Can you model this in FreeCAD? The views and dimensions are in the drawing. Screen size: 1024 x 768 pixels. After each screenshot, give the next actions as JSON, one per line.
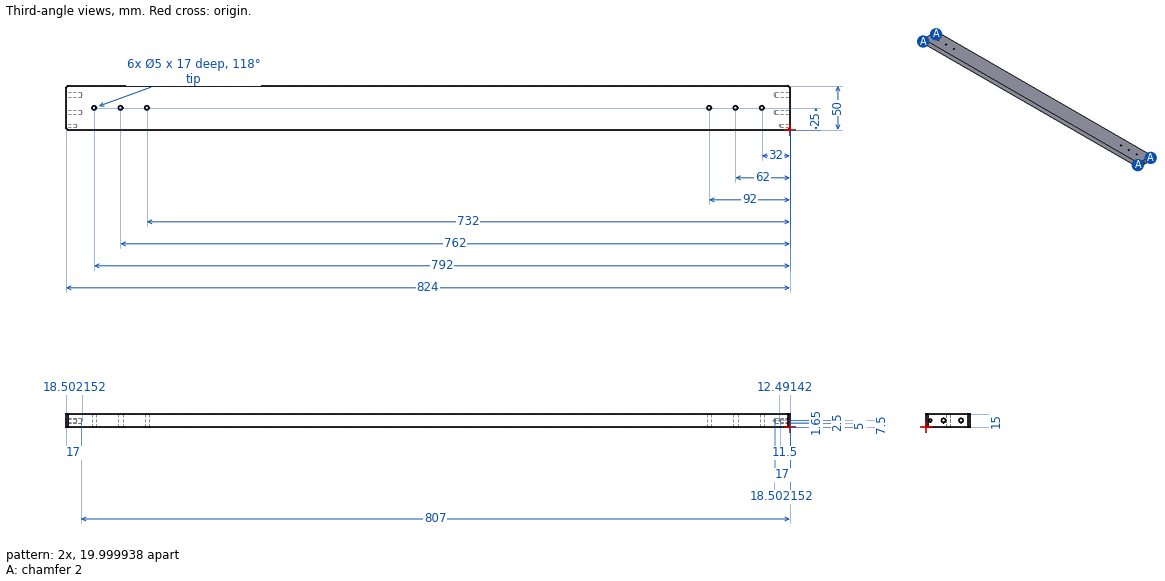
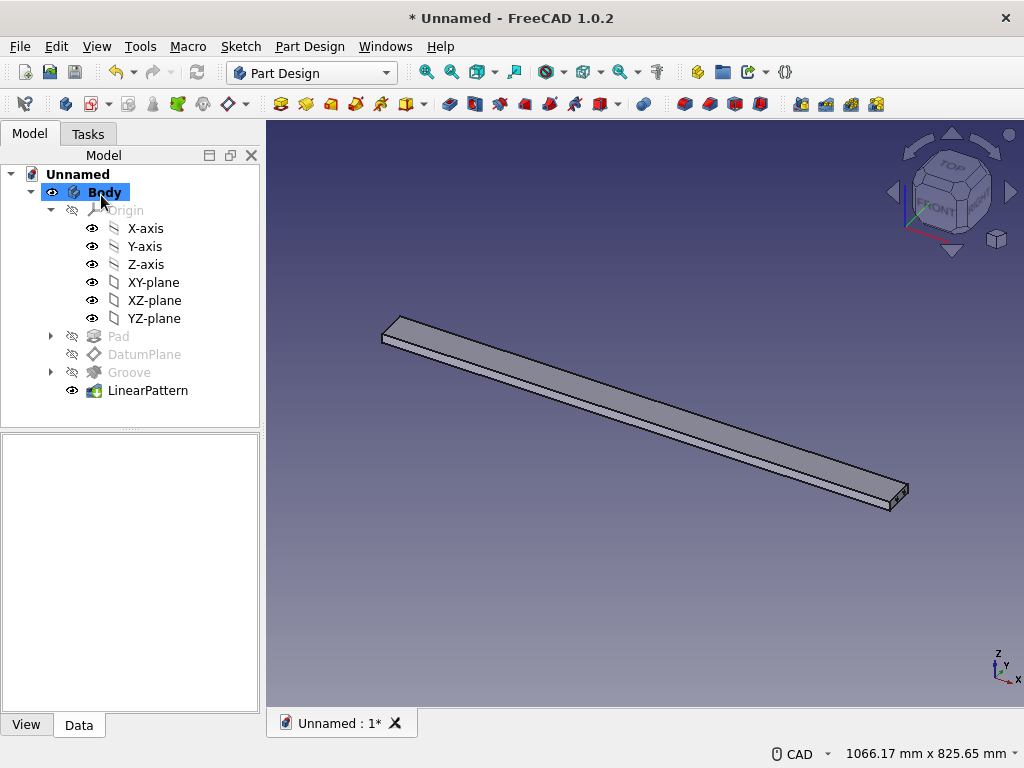
{"action": "left_click", "coordinate": [137, 300]}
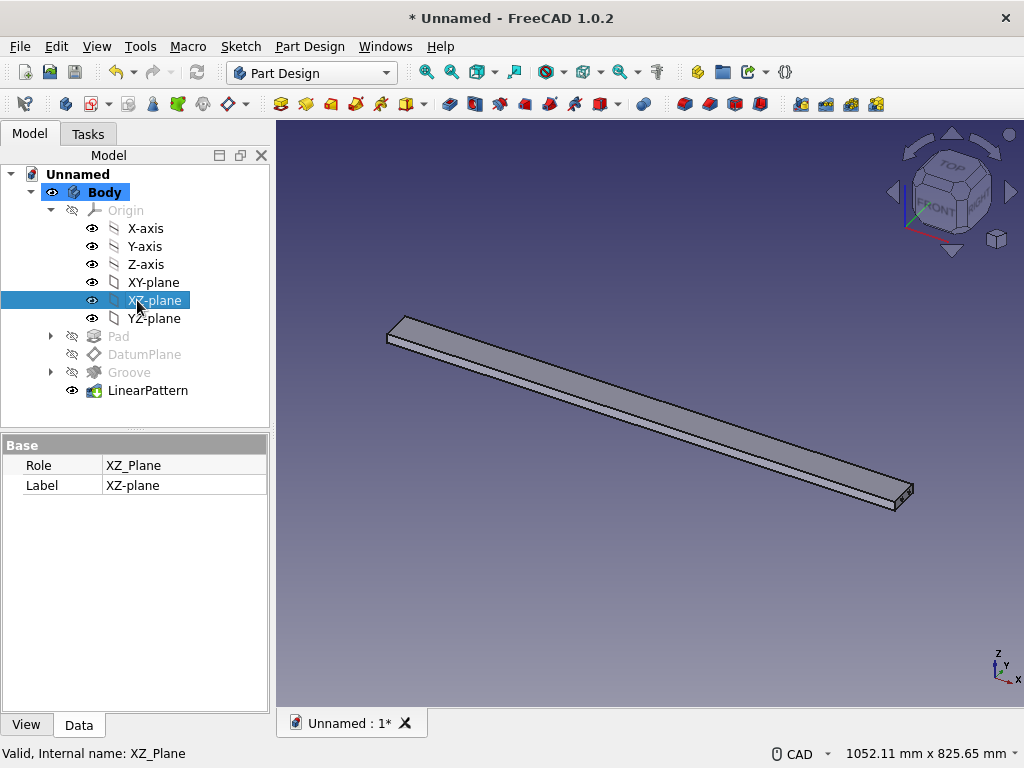
{"action": "left_click", "coordinate": [228, 104]}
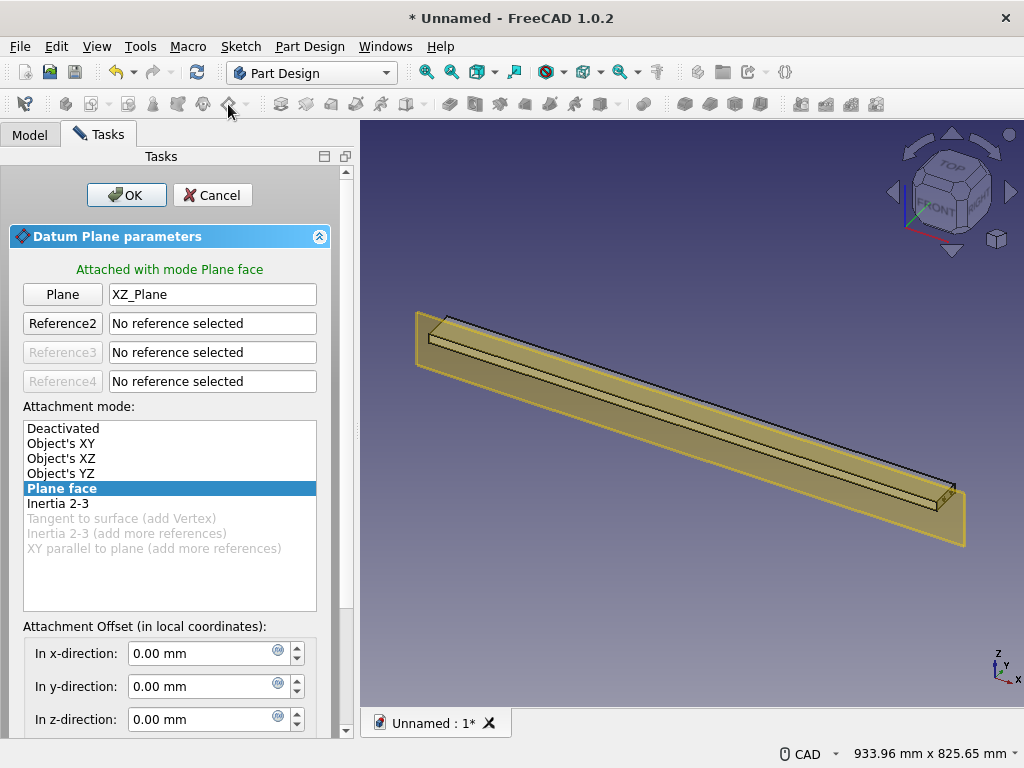
{"action": "triple_click", "coordinate": [210, 720]}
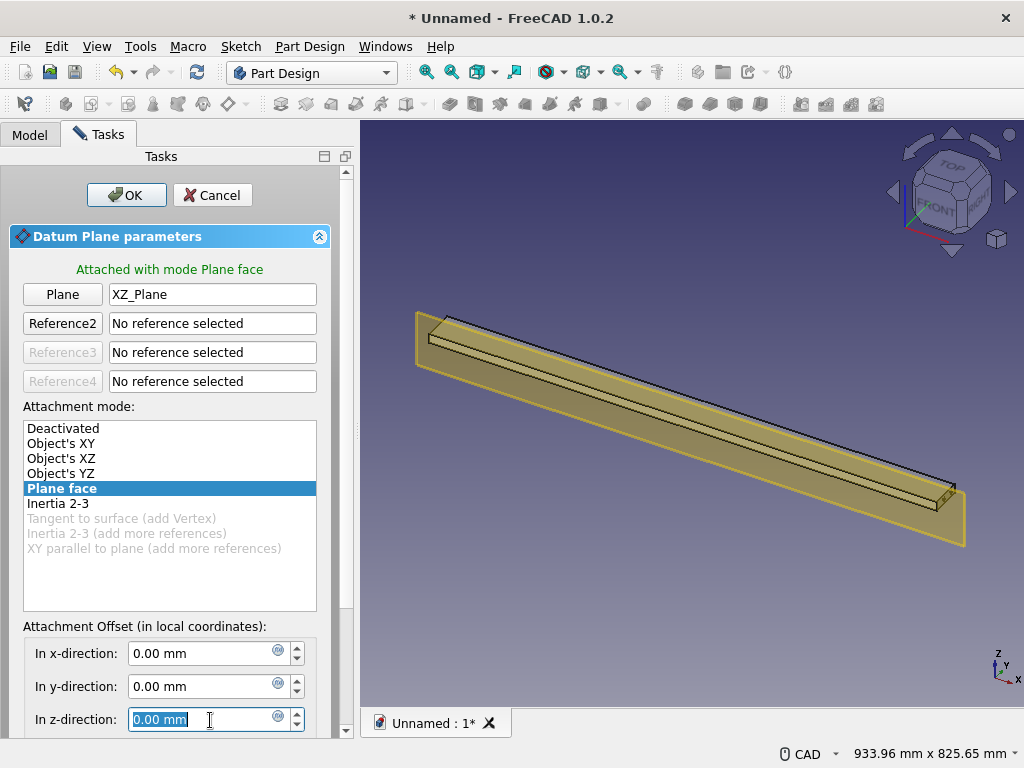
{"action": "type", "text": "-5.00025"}
{"action": "key", "text": "Tab"}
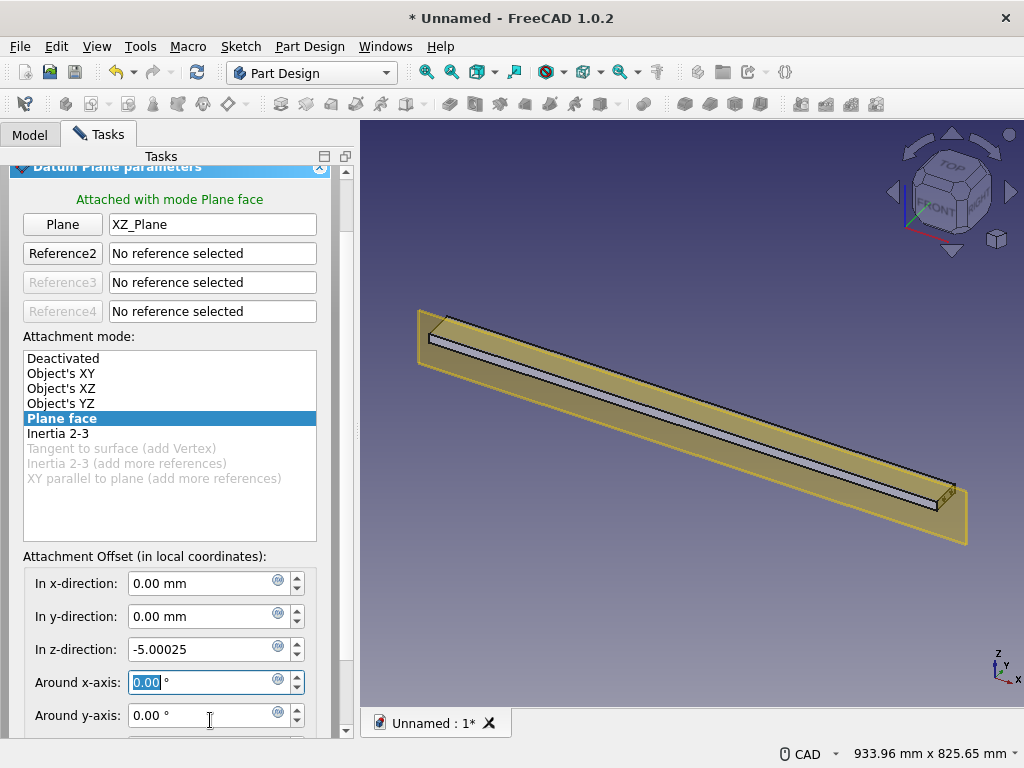
{"action": "scroll", "coordinate": [346, 452], "scroll_direction": "up", "scroll_amount": 2}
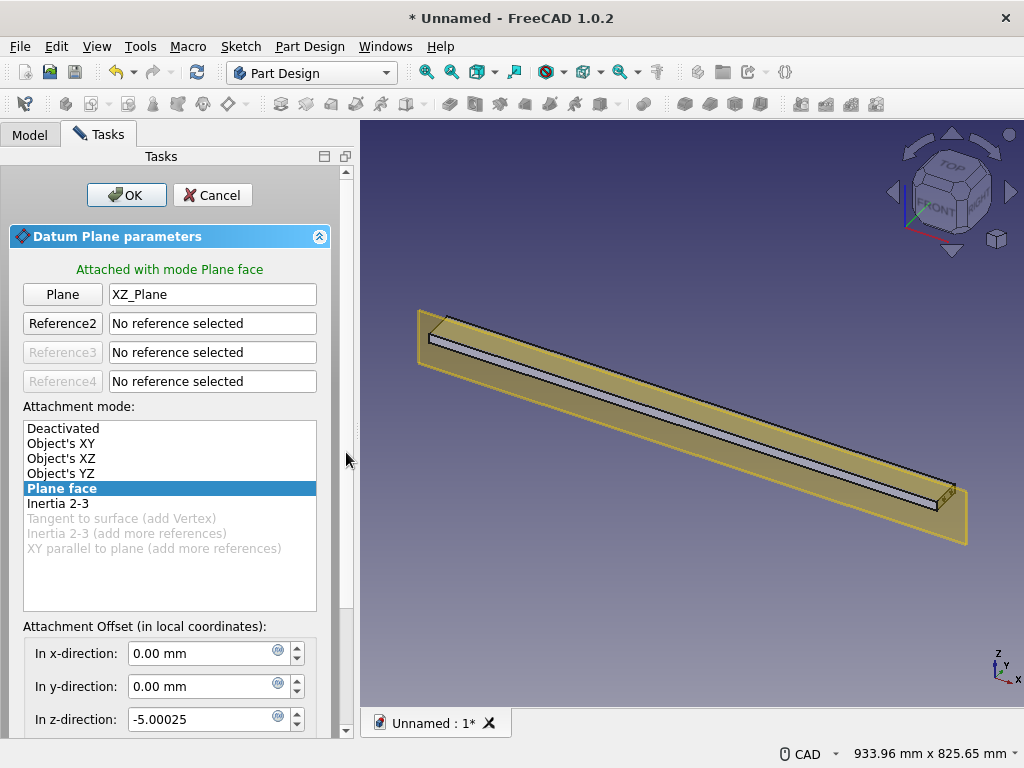
{"action": "left_click", "coordinate": [127, 195]}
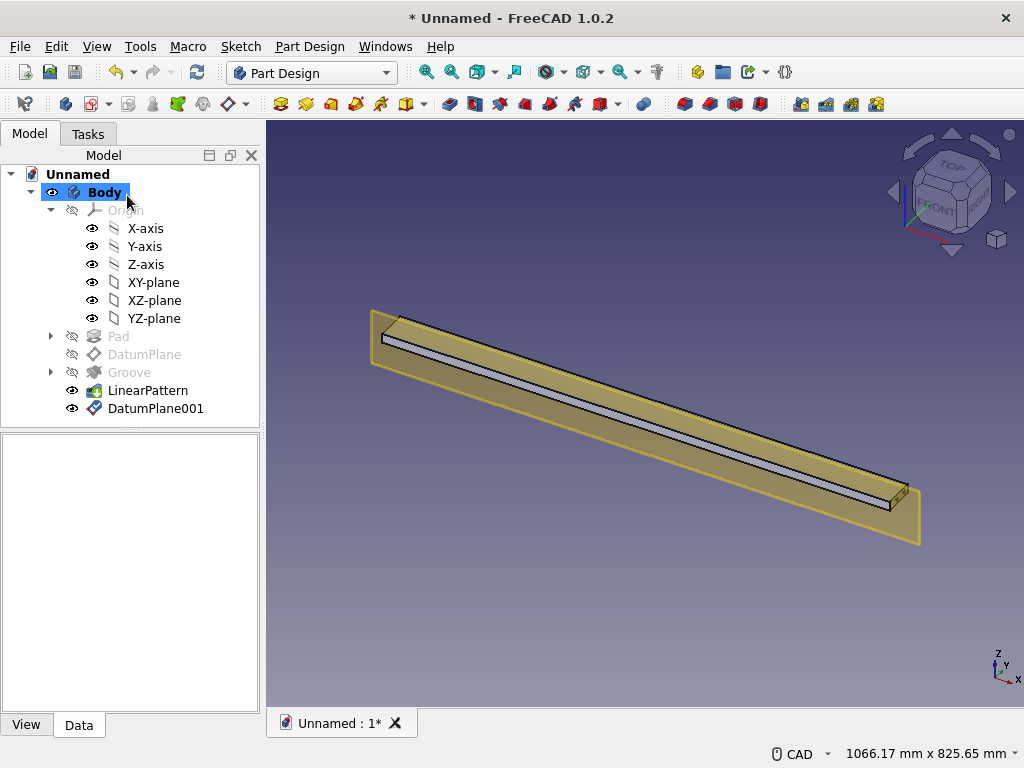
{"action": "left_click", "coordinate": [117, 408]}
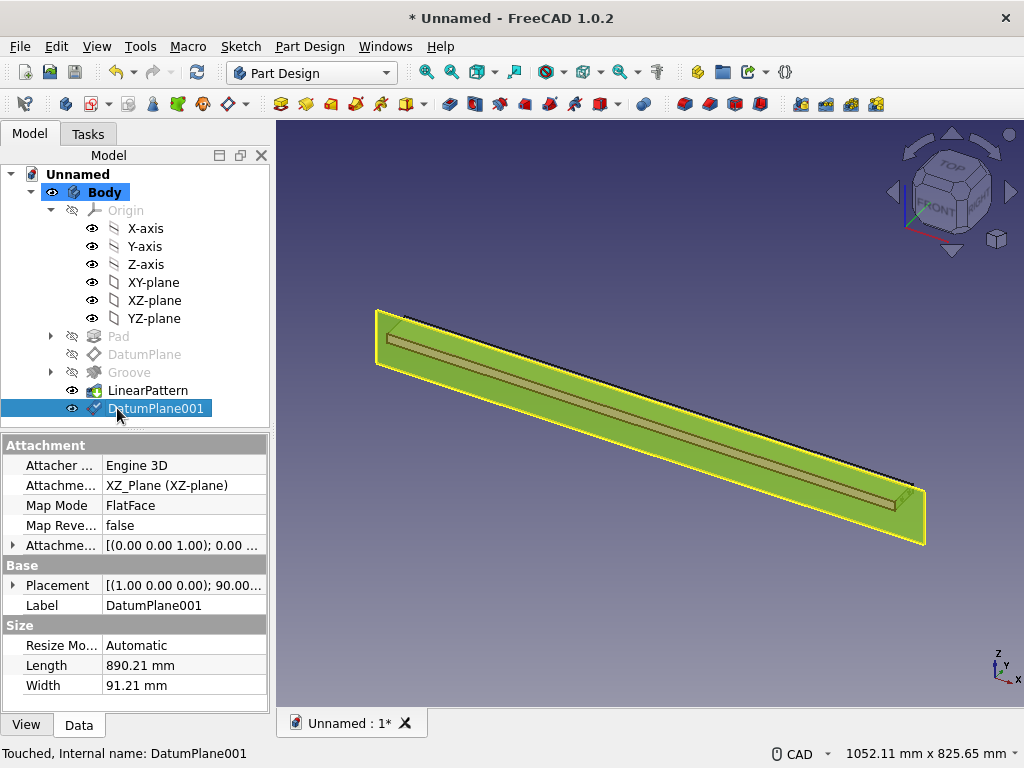
{"action": "left_click", "coordinate": [90, 104]}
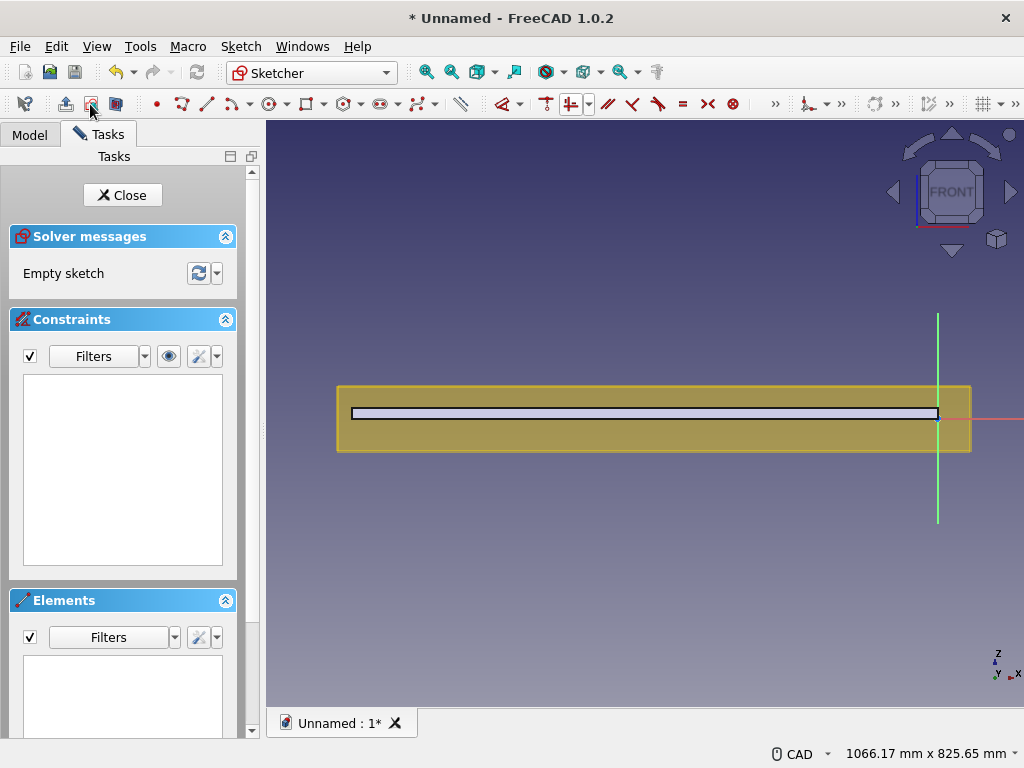
{"action": "left_click", "coordinate": [116, 104]}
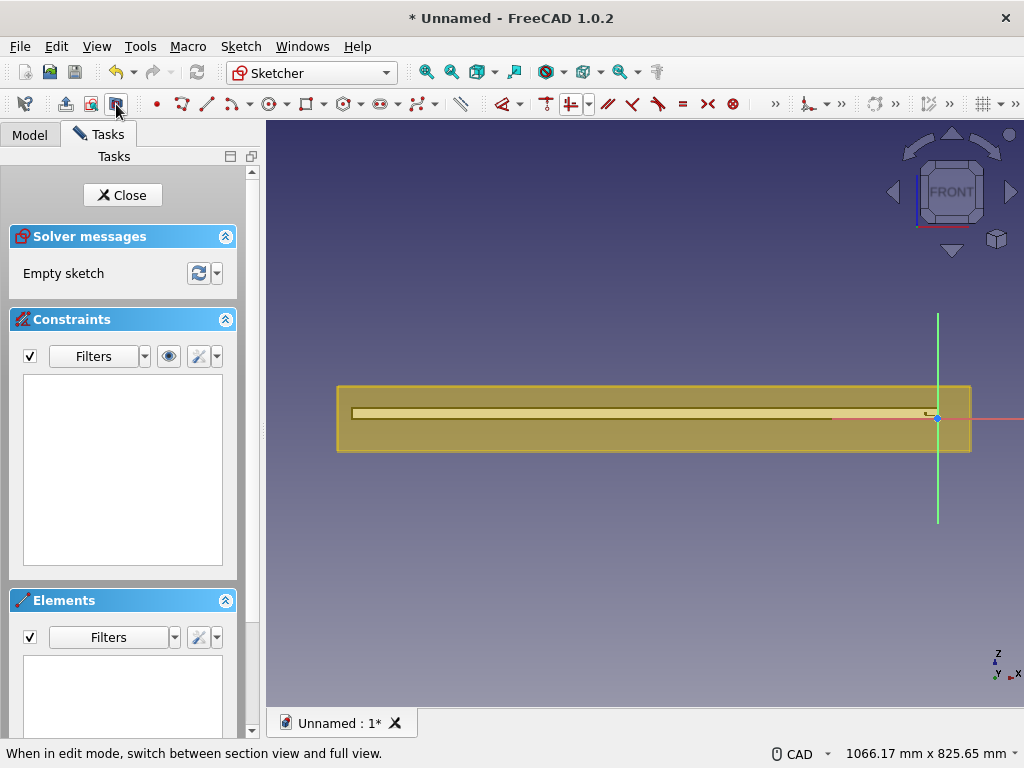
{"action": "scroll", "coordinate": [576, 414], "scroll_direction": "down", "scroll_amount": 5}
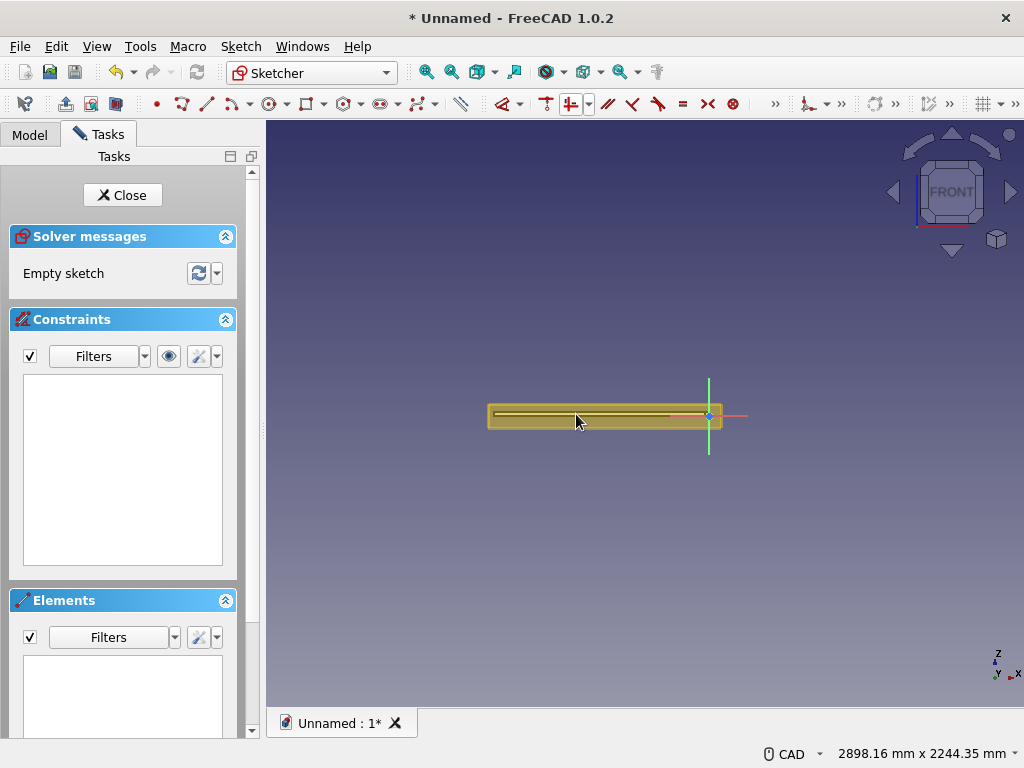
{"action": "scroll", "coordinate": [714, 415], "scroll_direction": "up", "scroll_amount": 15}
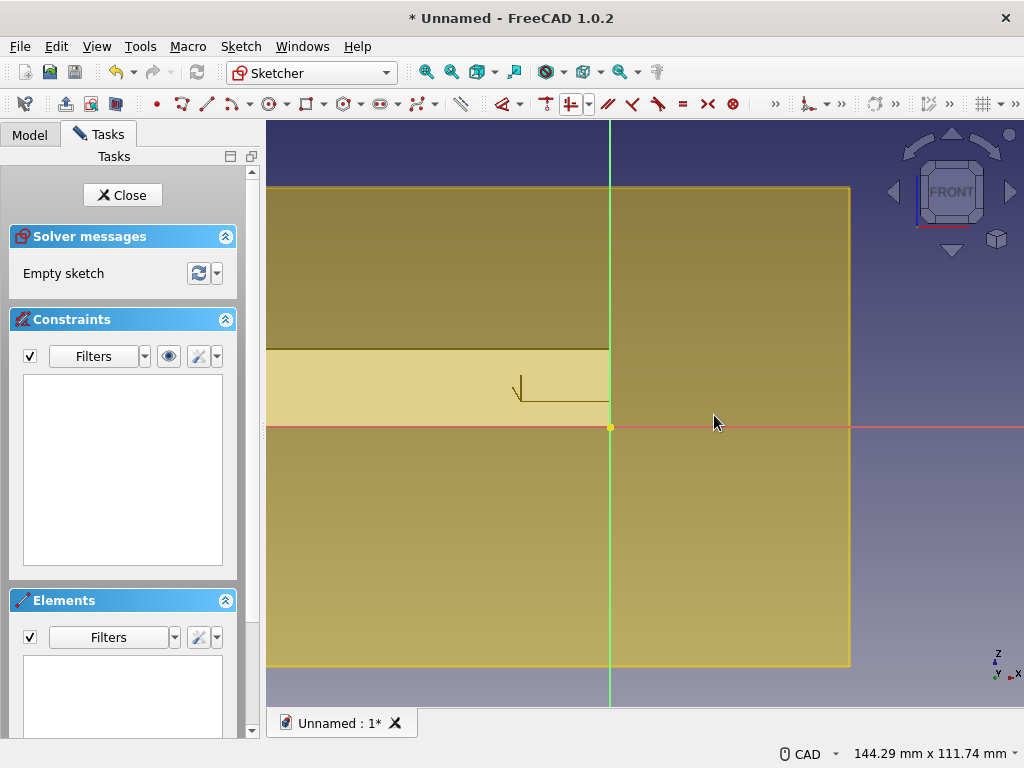
{"action": "scroll", "coordinate": [560, 406], "scroll_direction": "up", "scroll_amount": 7}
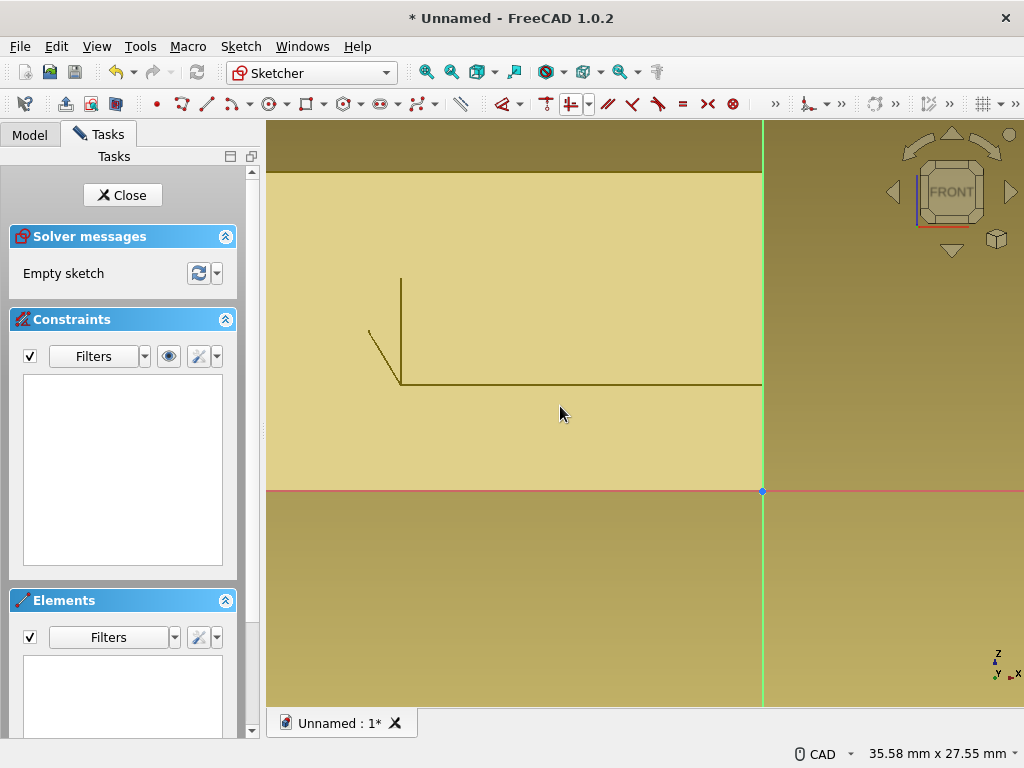
{"action": "left_click", "coordinate": [182, 104]}